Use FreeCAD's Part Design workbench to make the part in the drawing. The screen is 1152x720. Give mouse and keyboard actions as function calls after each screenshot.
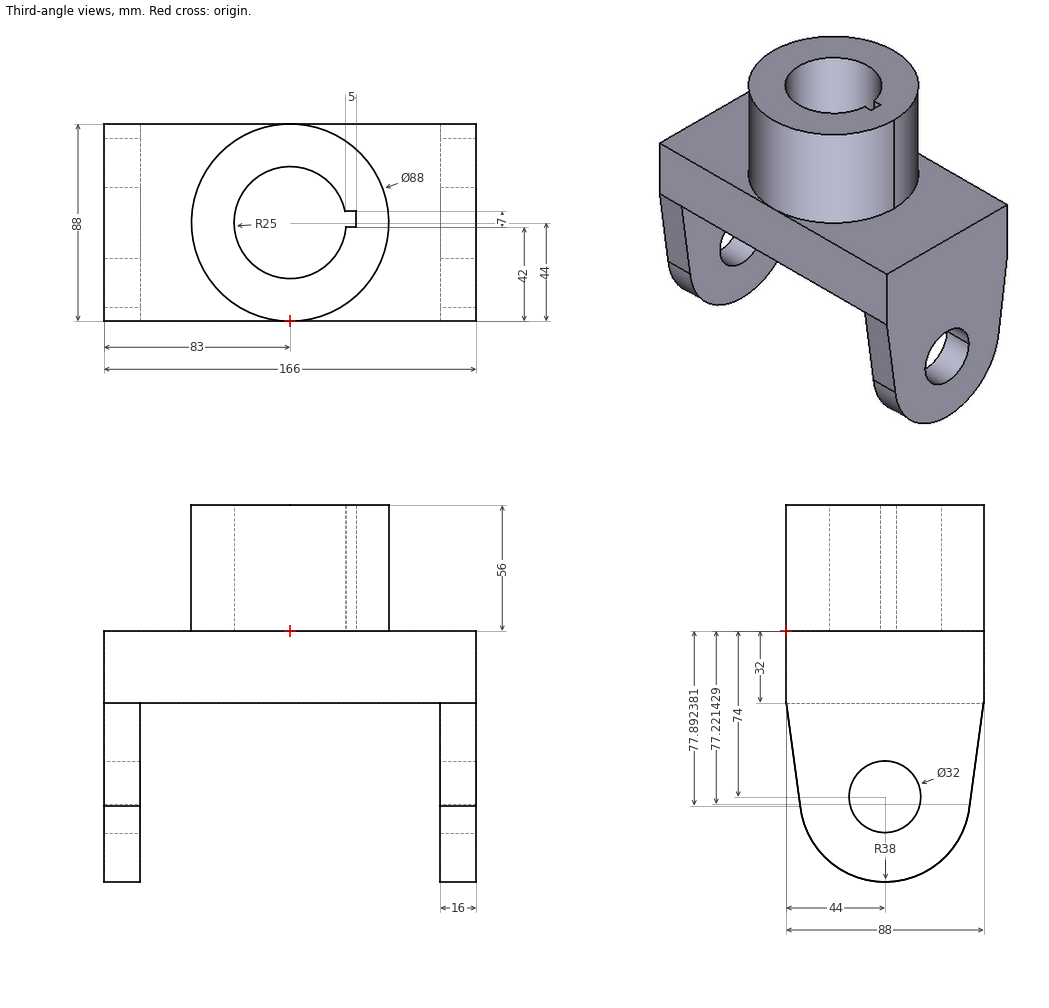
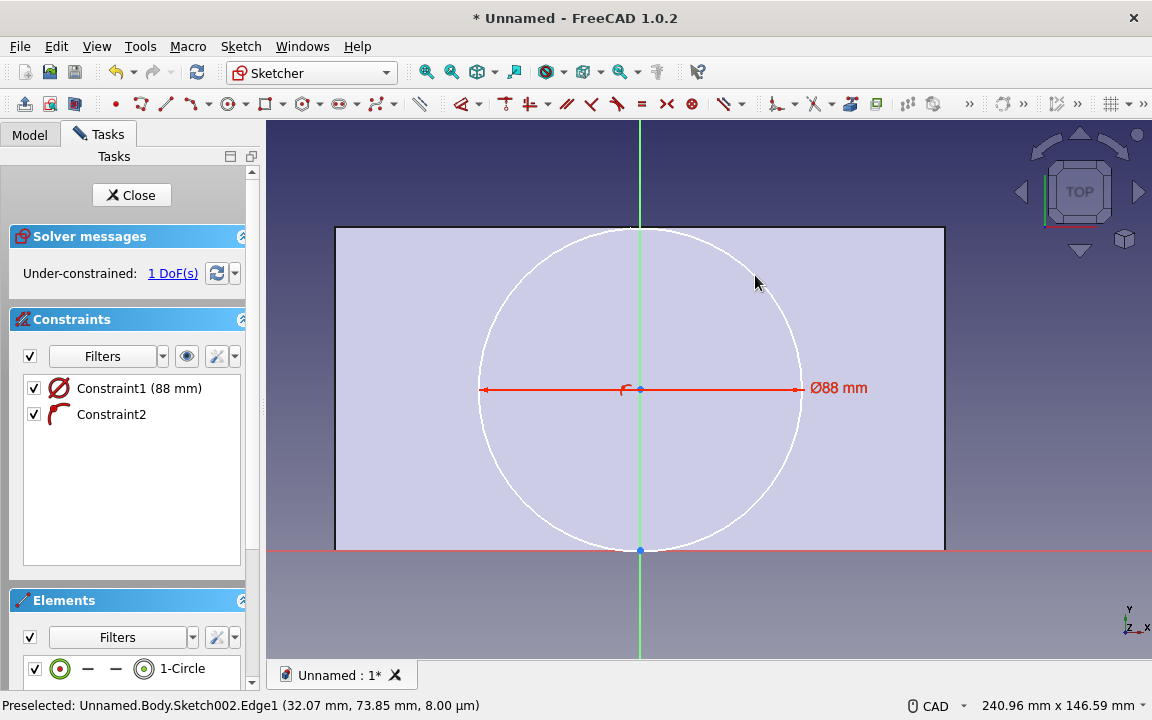
click(460, 104)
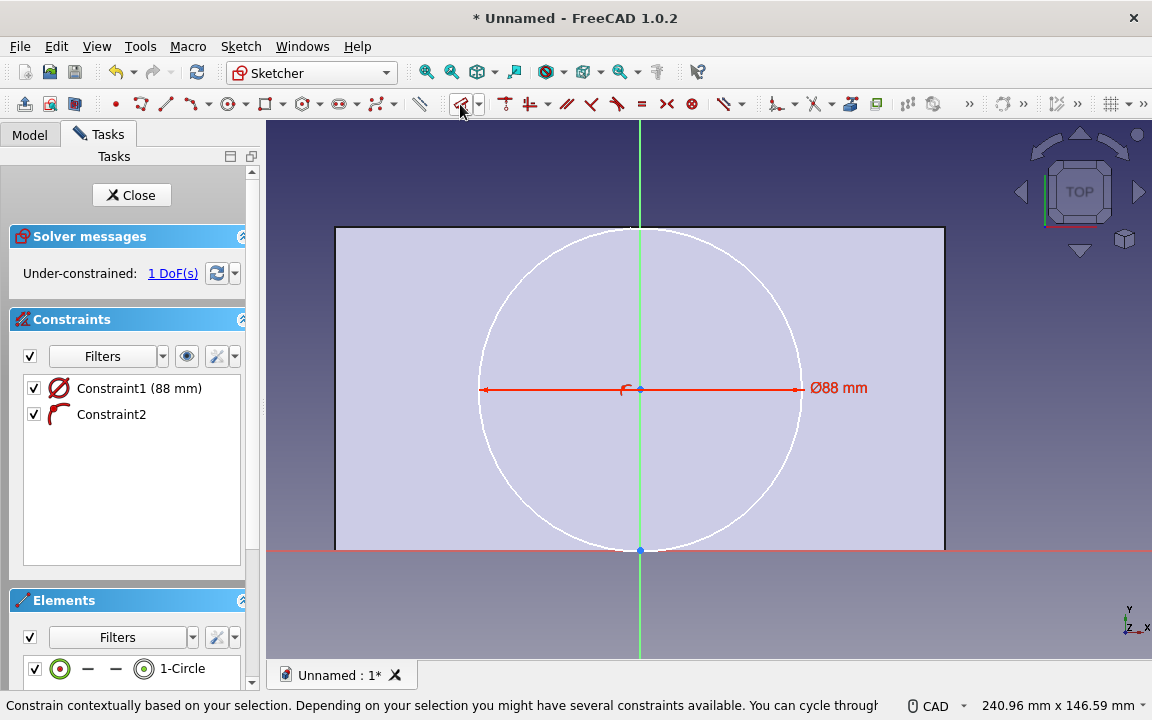
click(640, 390)
click(674, 470)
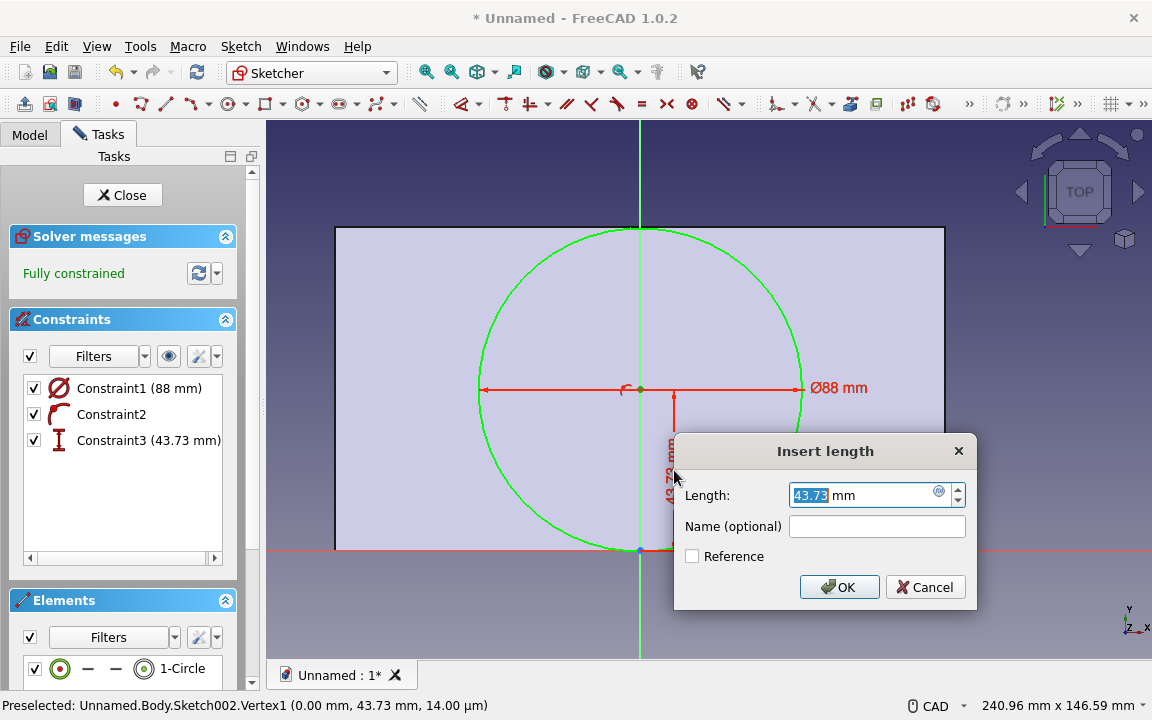
text(44)
key(Return)
key(Escape)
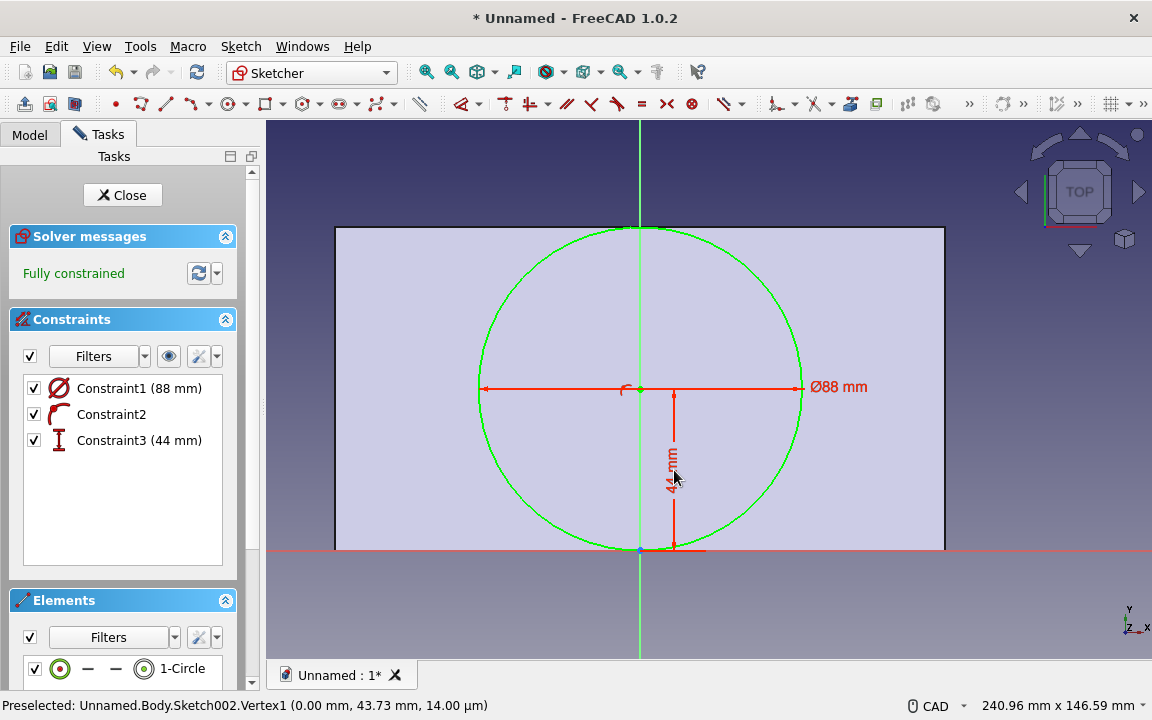
click(123, 195)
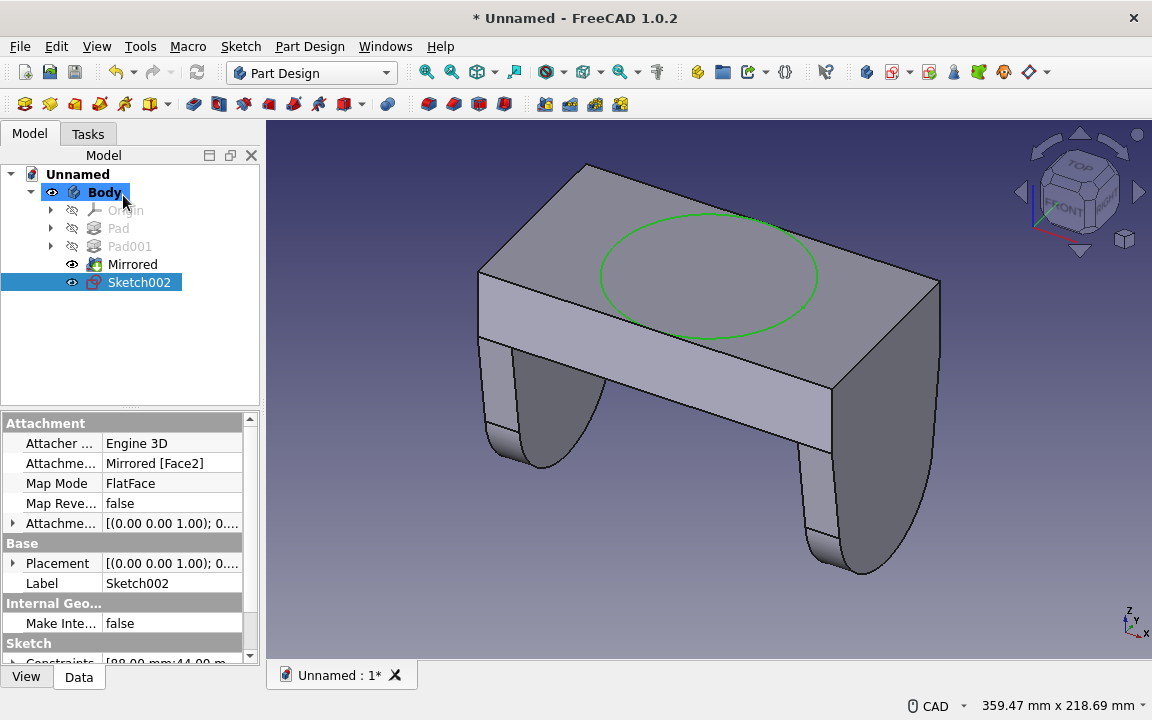
click(25, 104)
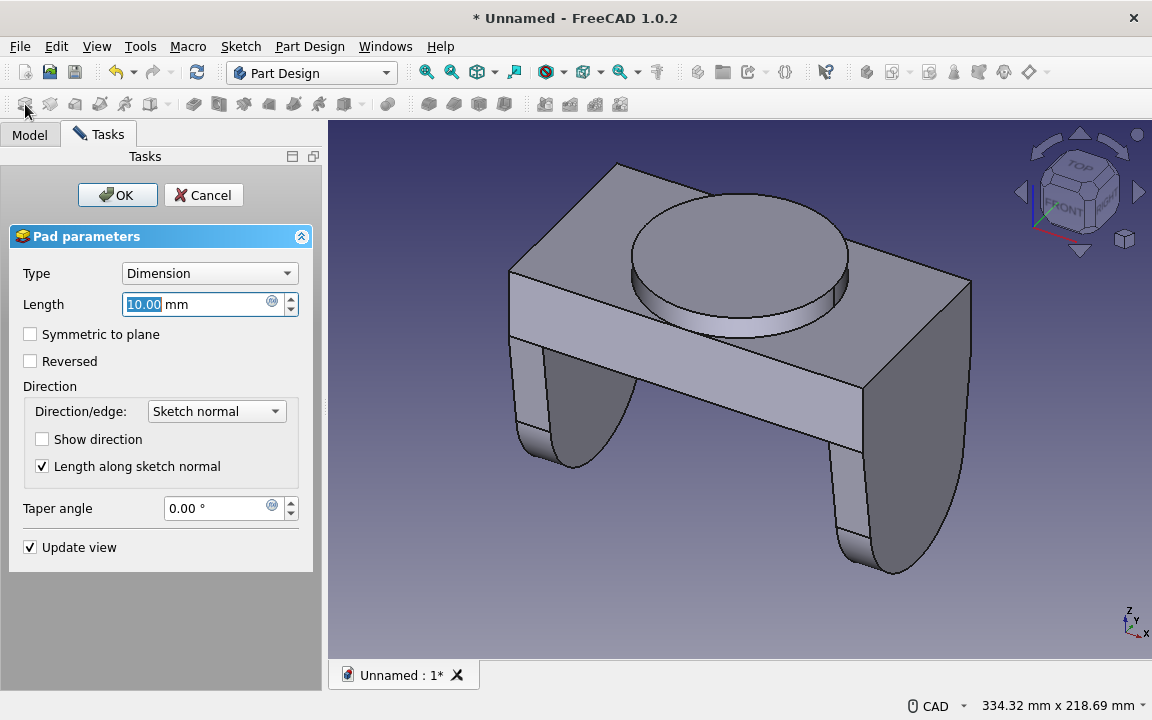
text(56)
key(Tab)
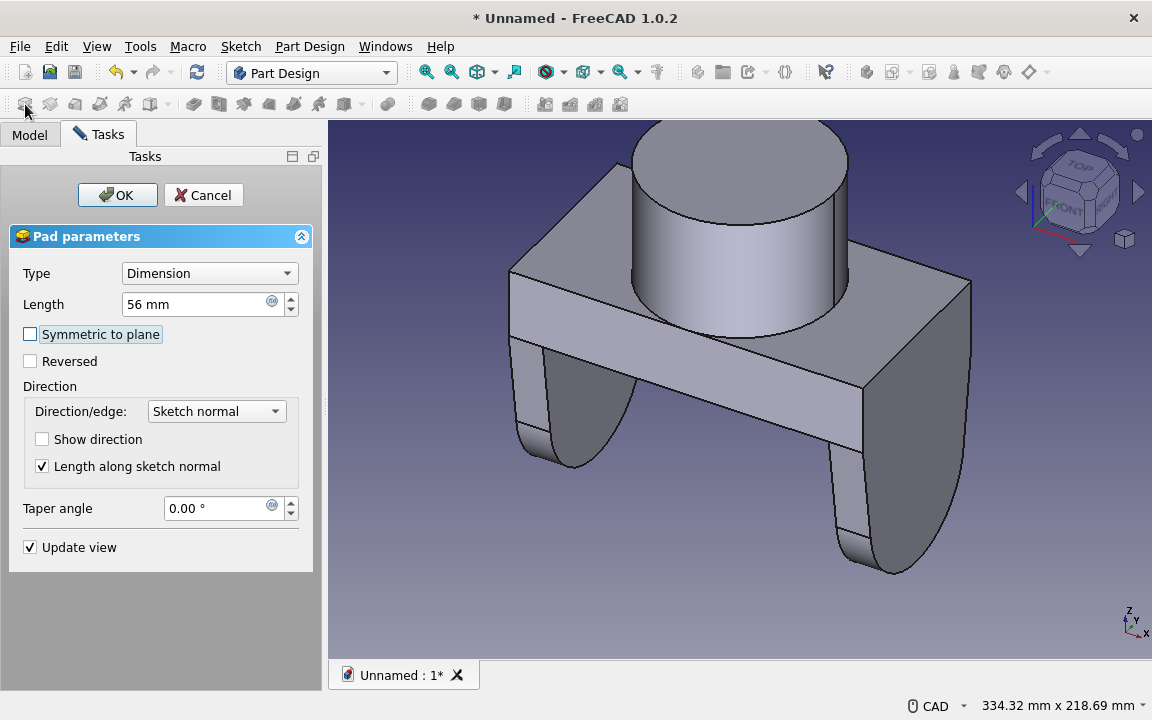
click(118, 195)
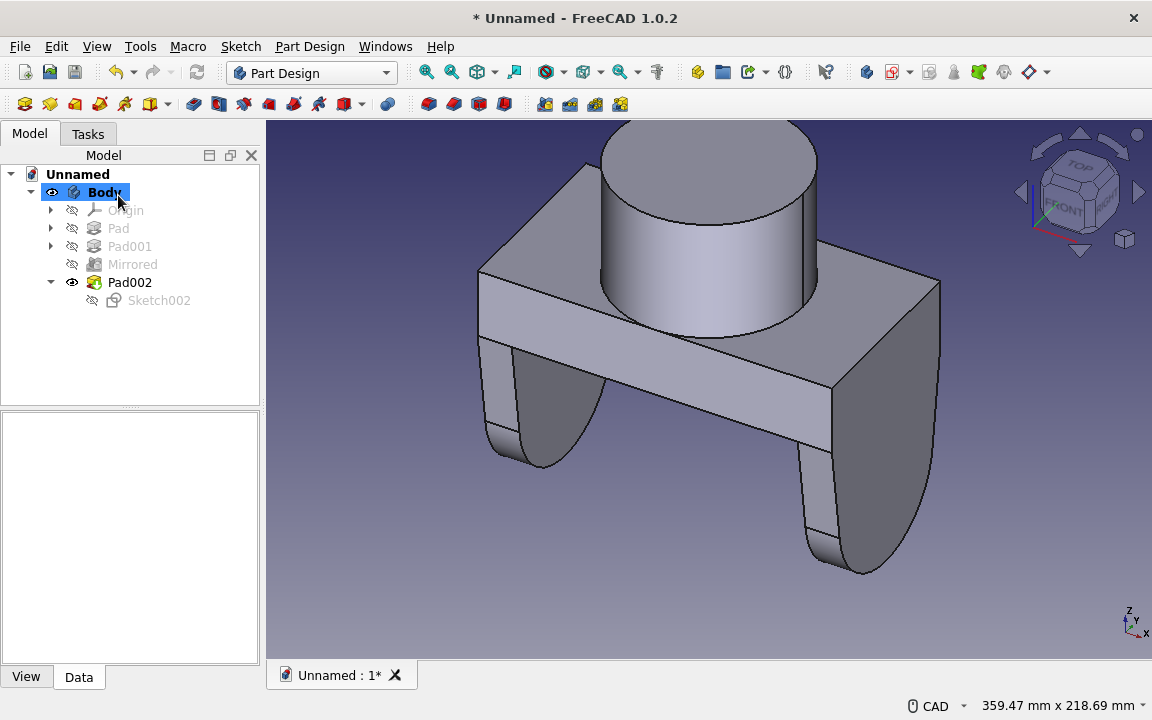
click(427, 72)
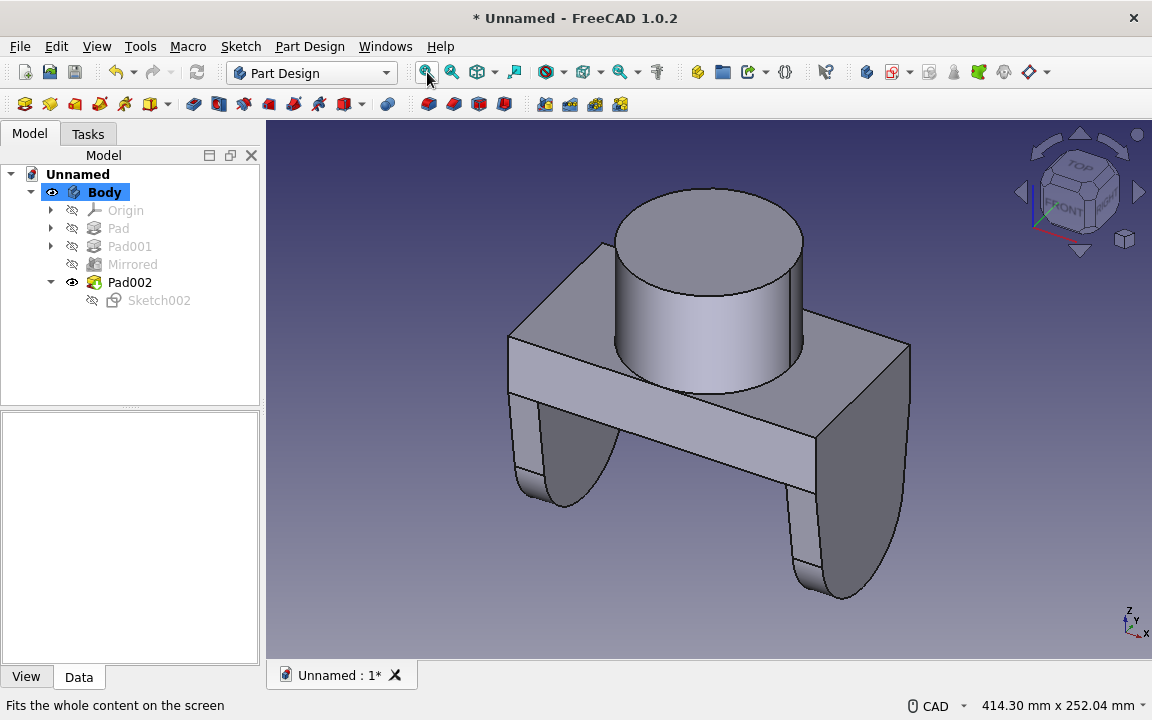
click(709, 241)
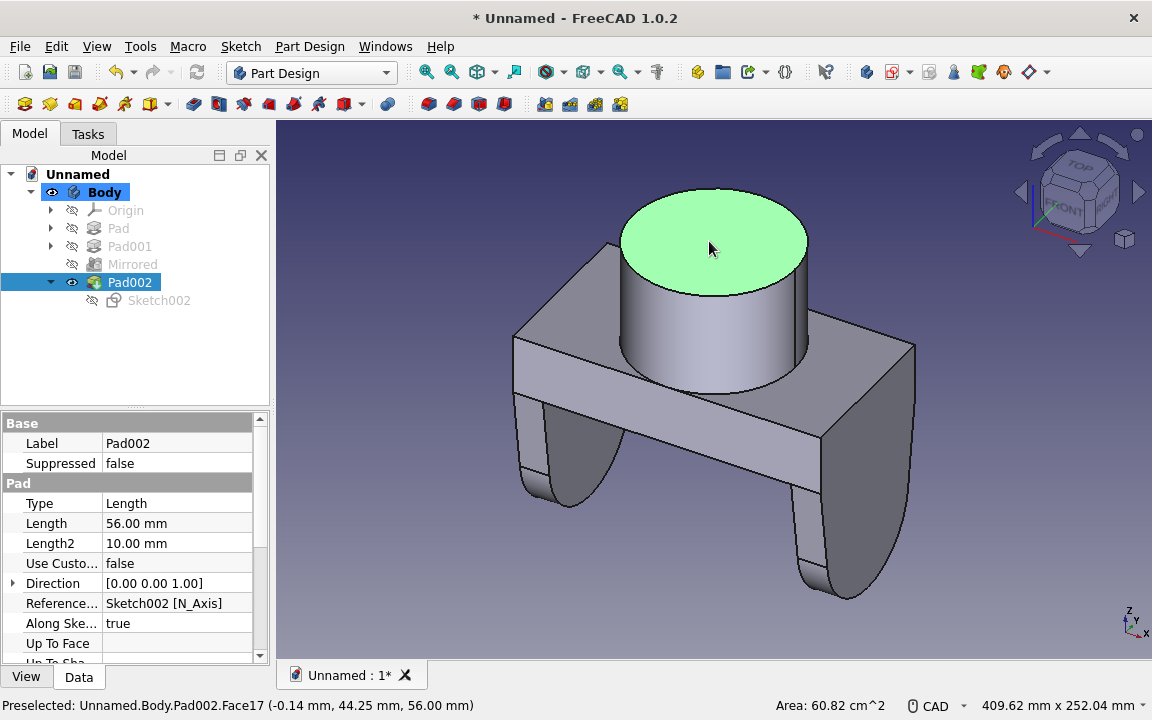
click(892, 72)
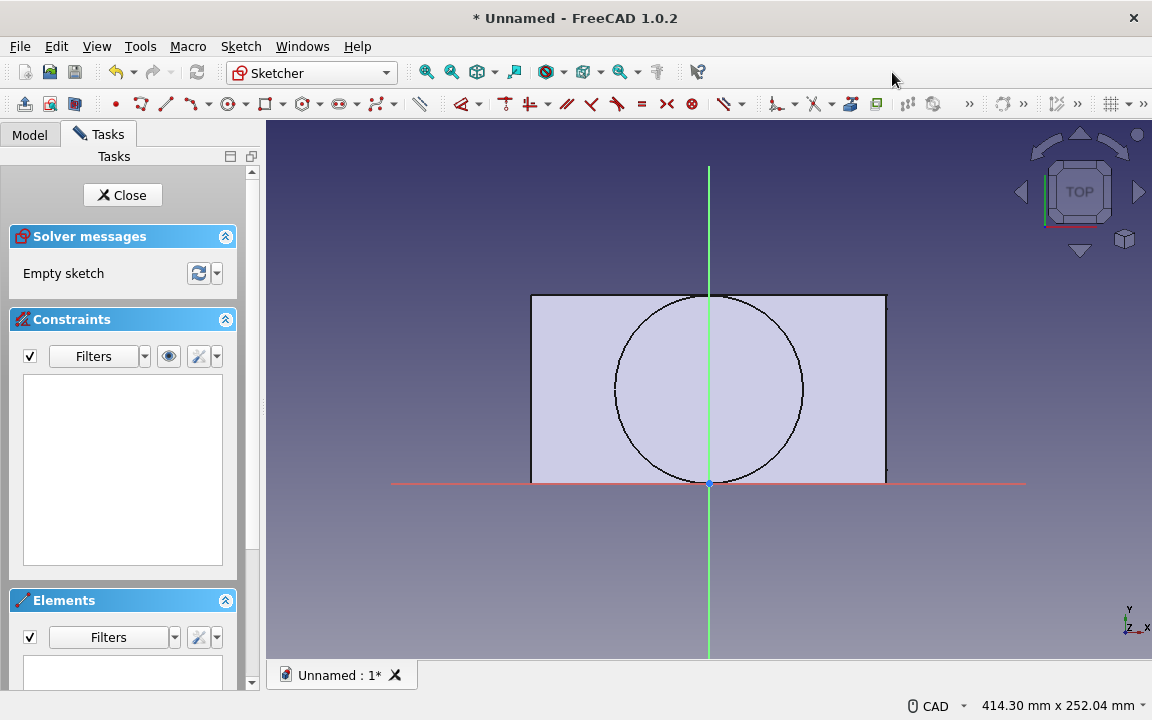
scroll(745, 449, up, 6)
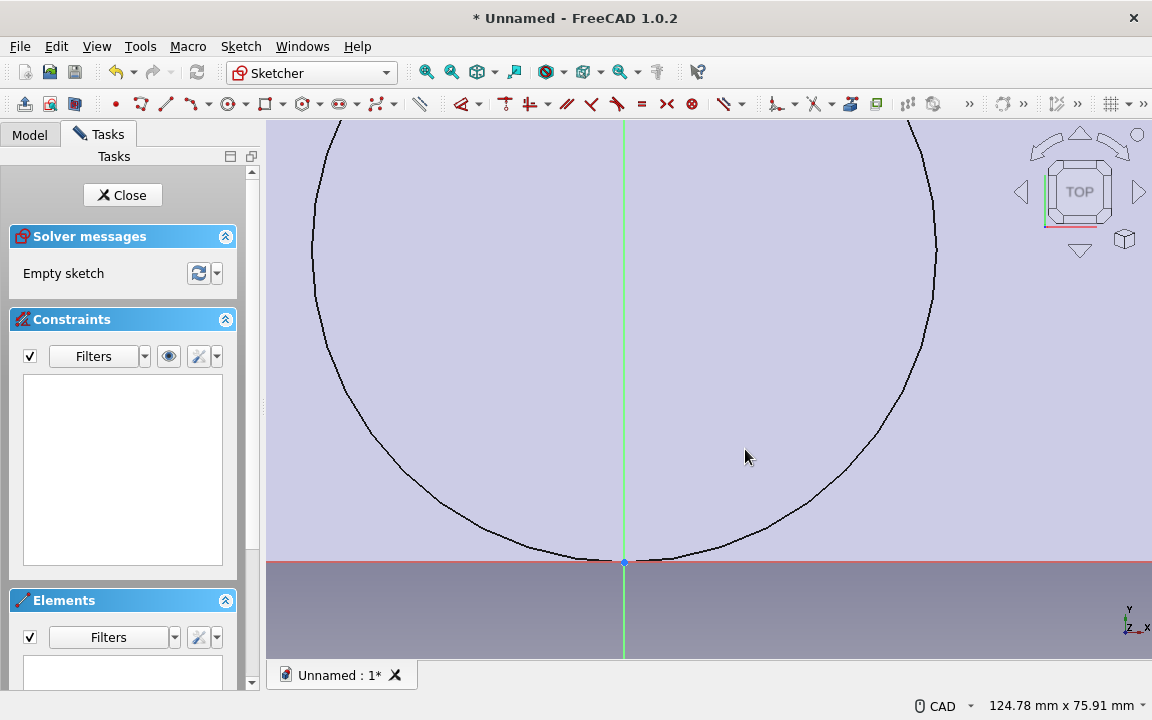
click(141, 104)